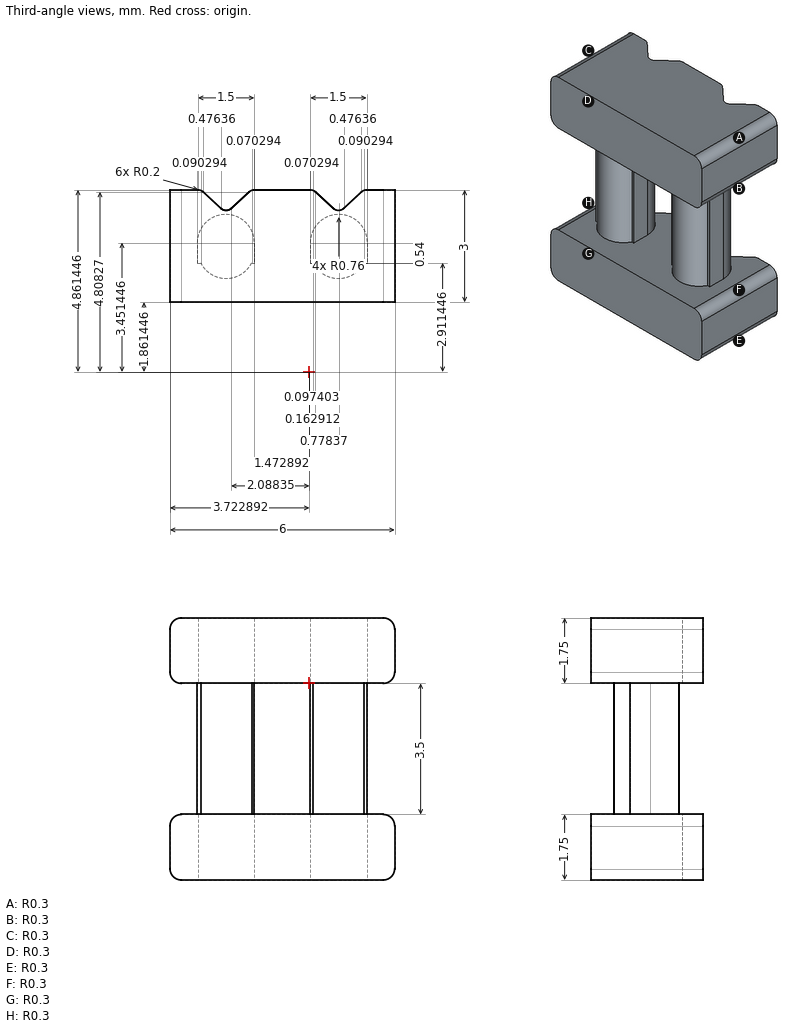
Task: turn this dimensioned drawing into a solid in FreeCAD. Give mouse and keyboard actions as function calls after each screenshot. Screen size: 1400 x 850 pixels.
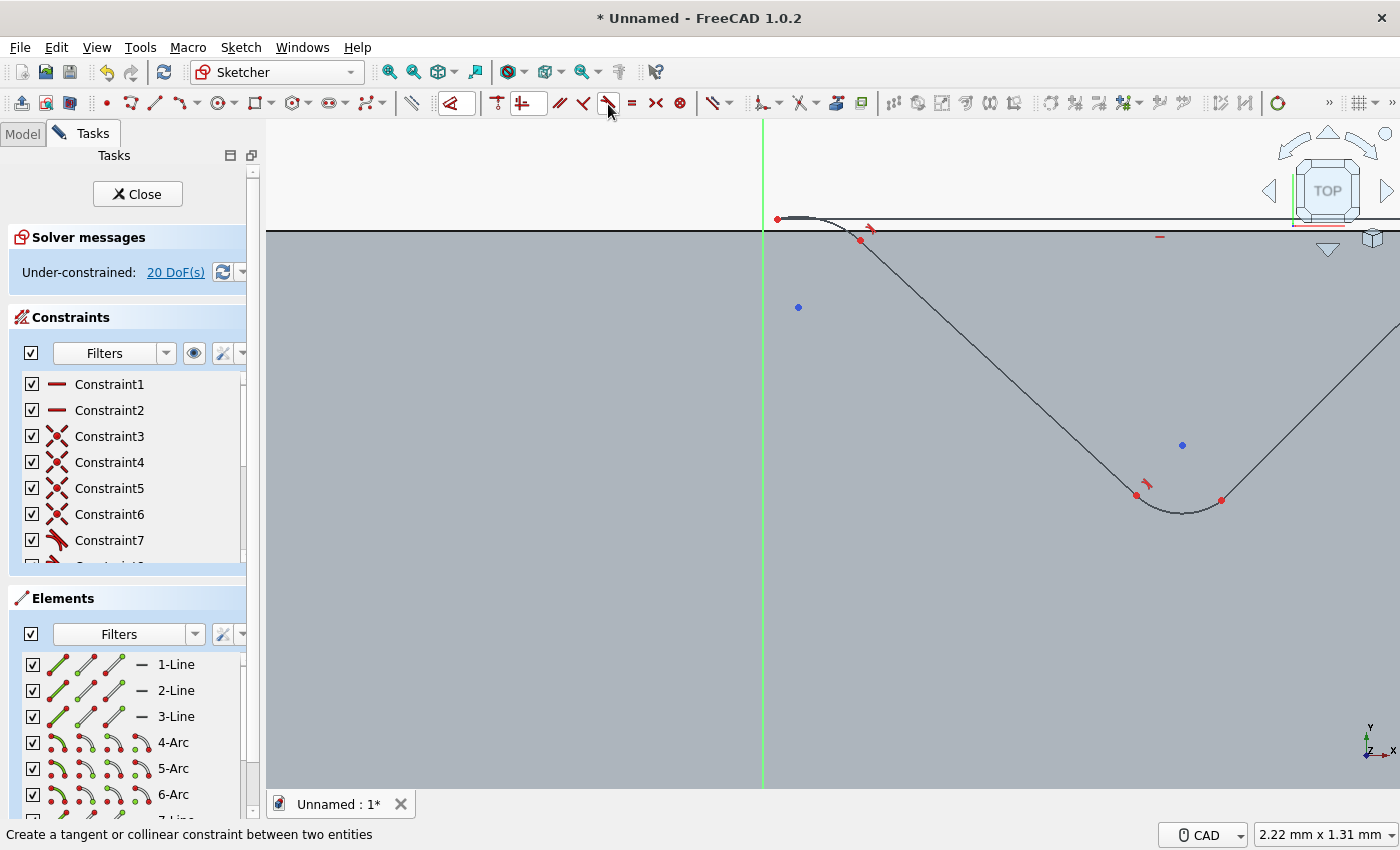
scroll(838, 252, down, 9)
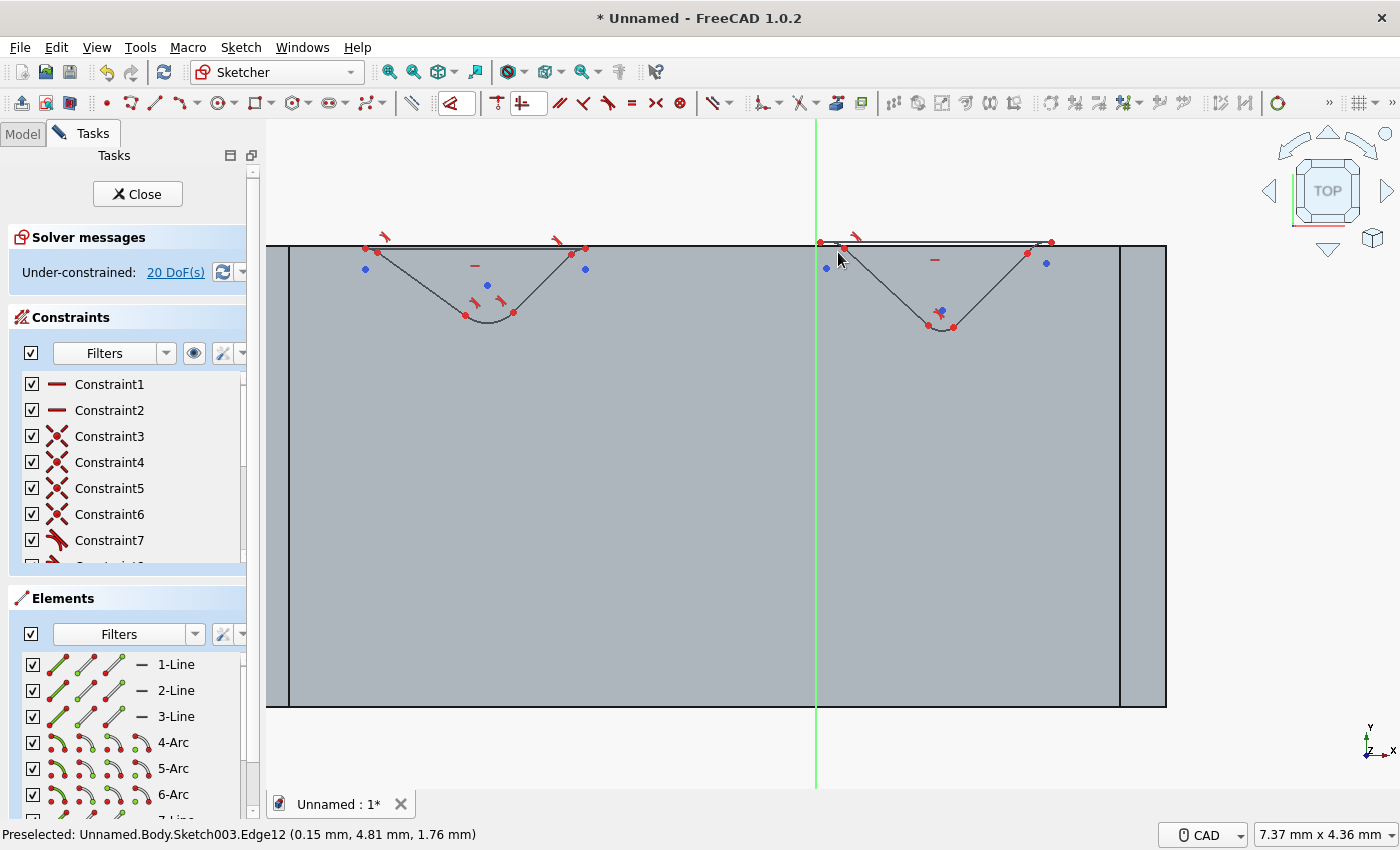
click(914, 281)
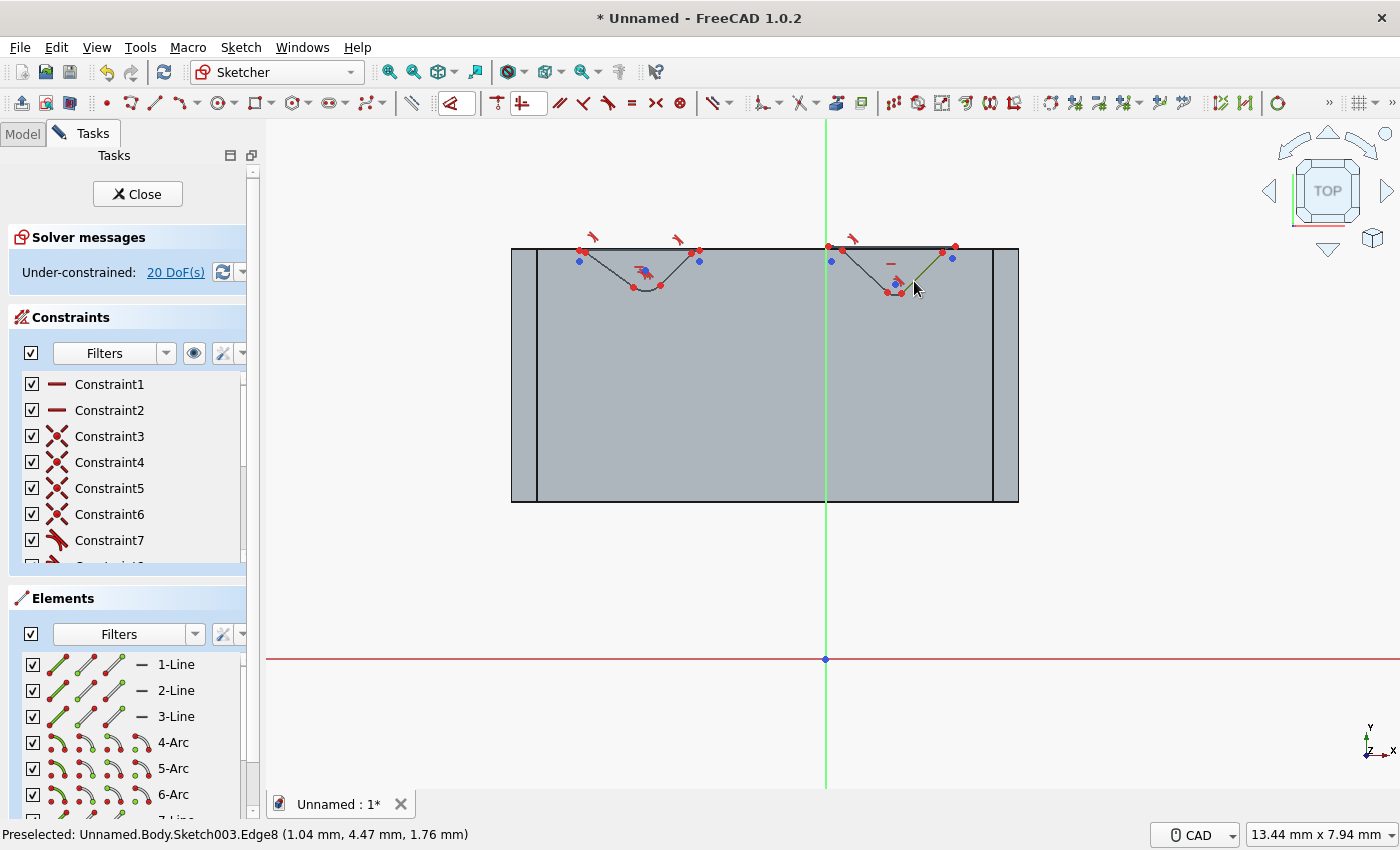
scroll(895, 295, up, 4)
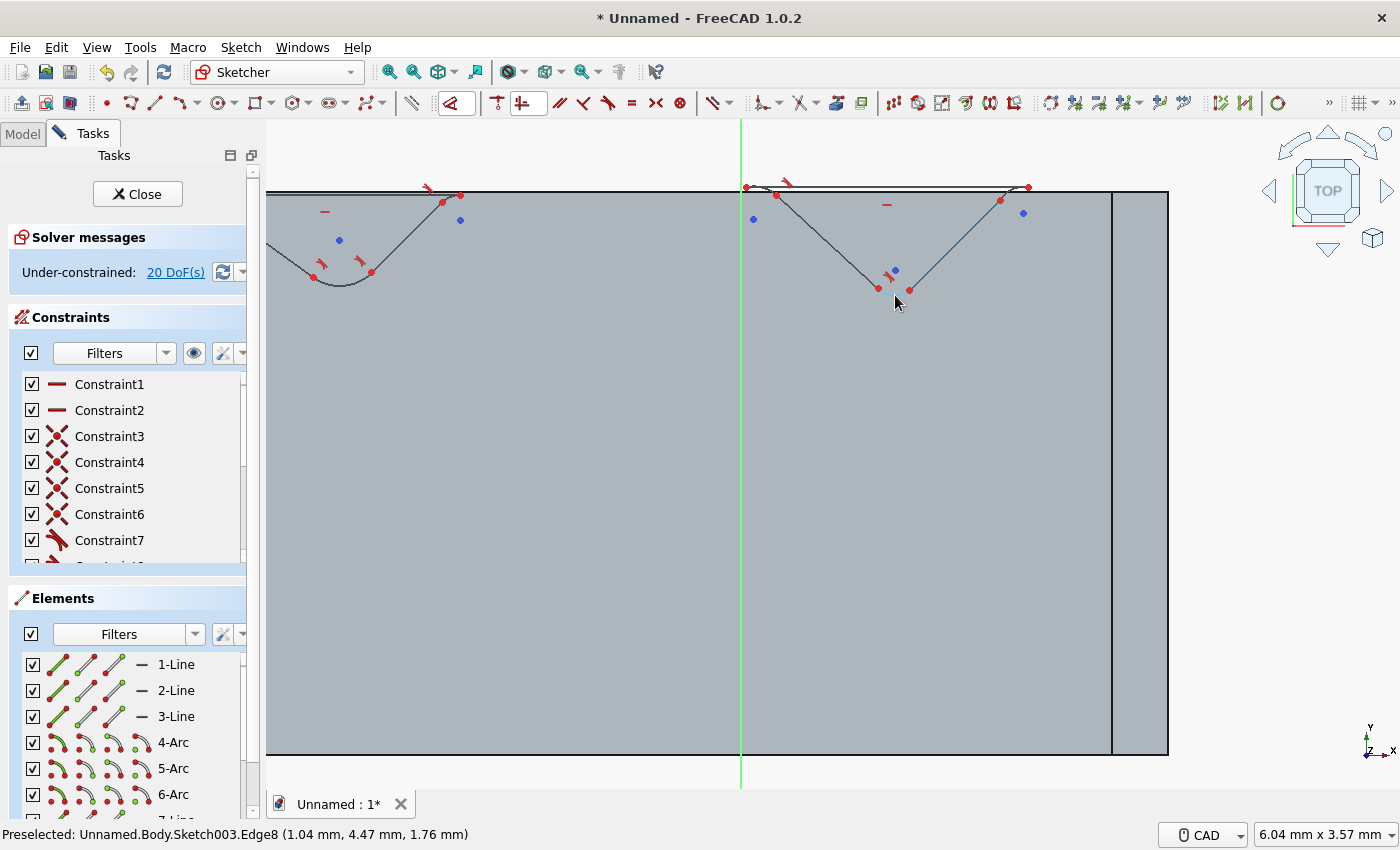
click(894, 296)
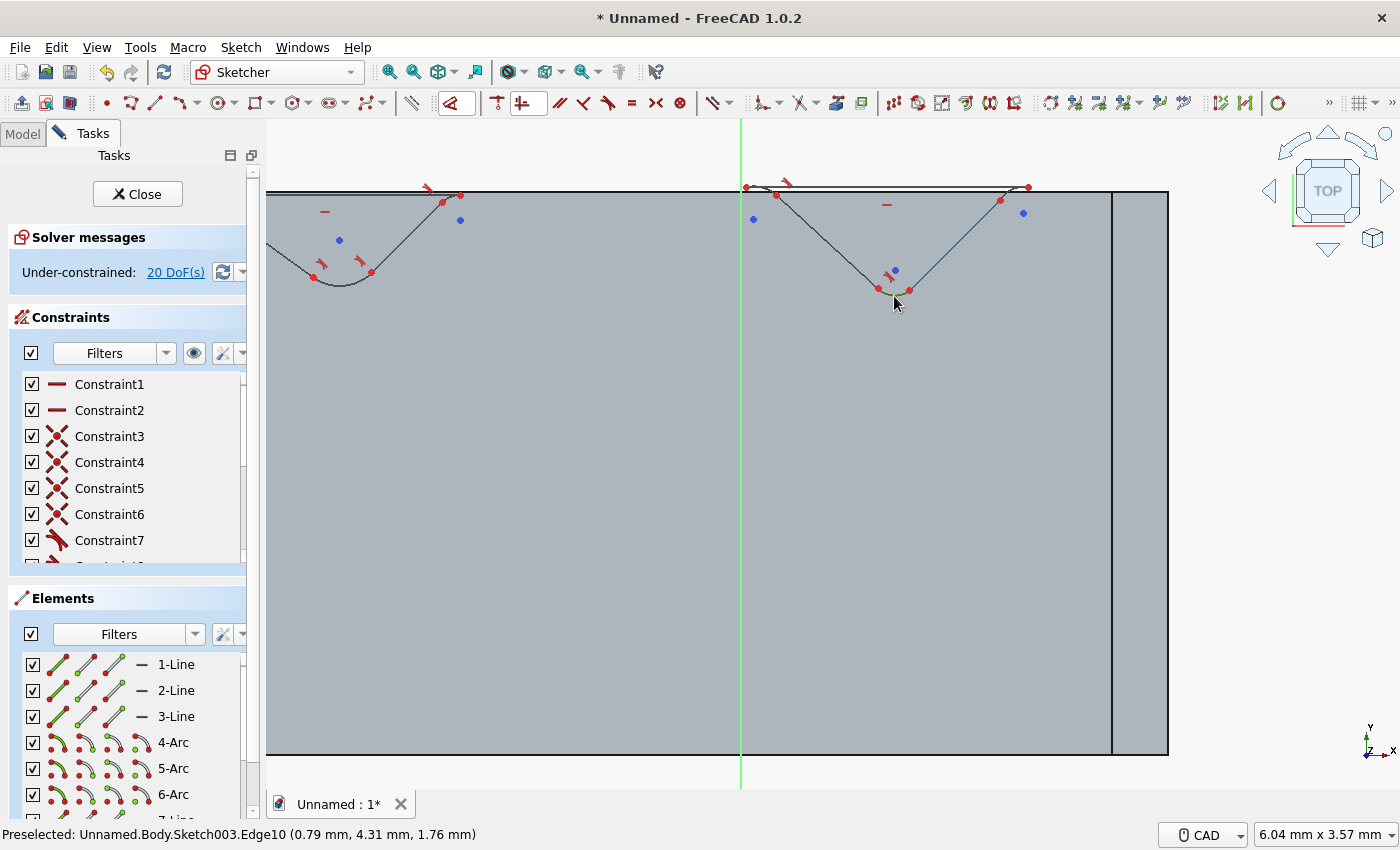
click(608, 104)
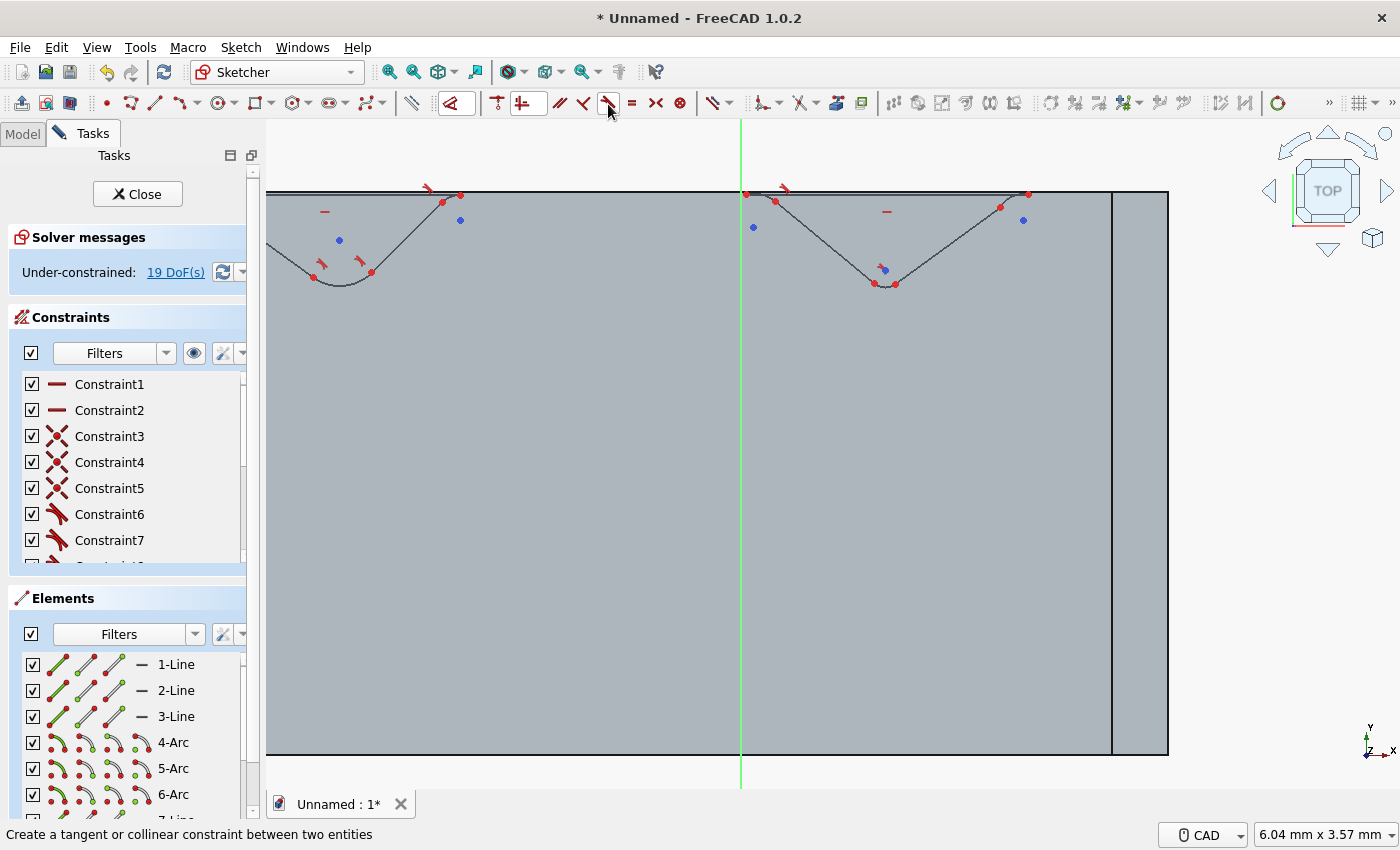
click(927, 261)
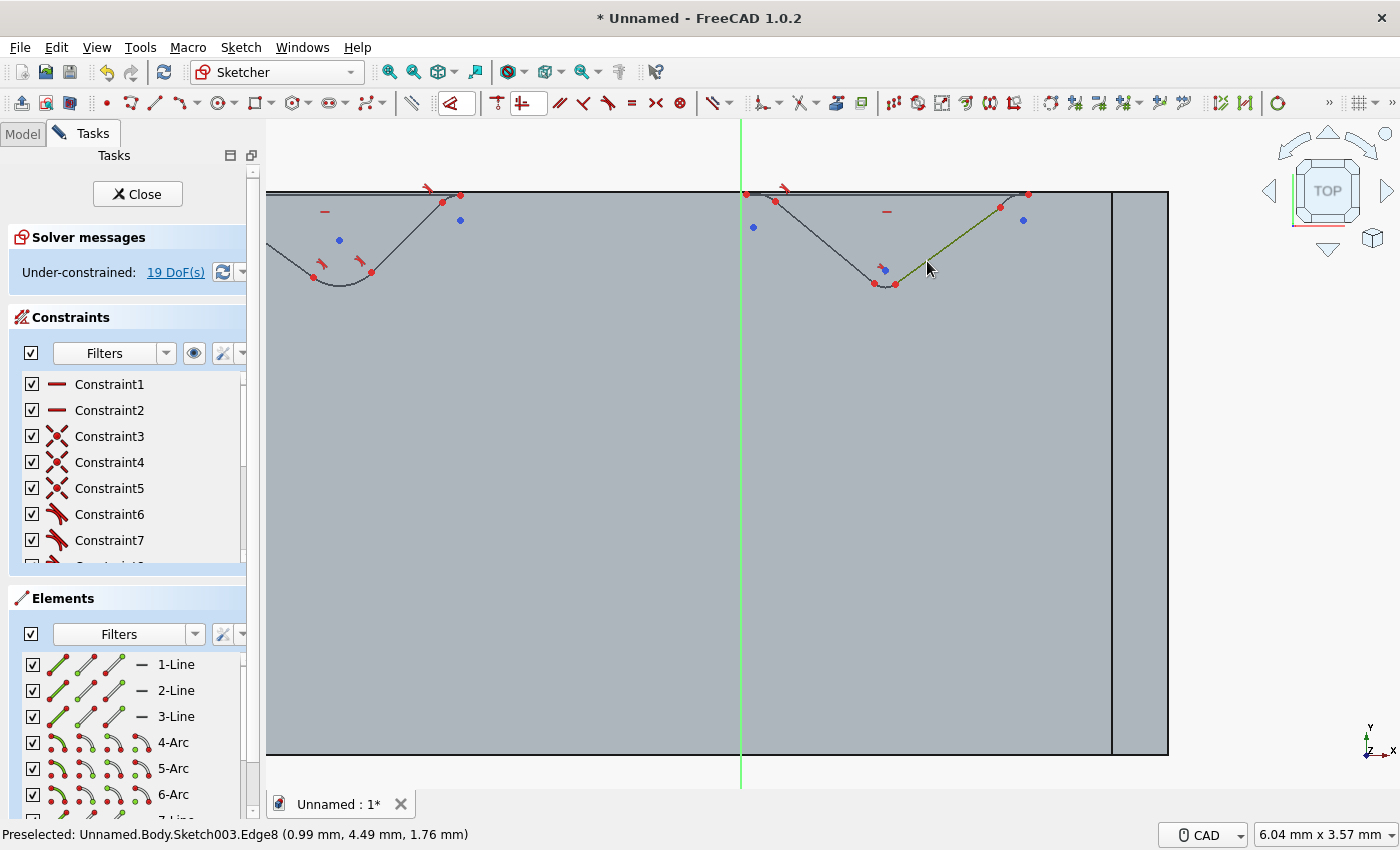
scroll(1004, 202, up, 4)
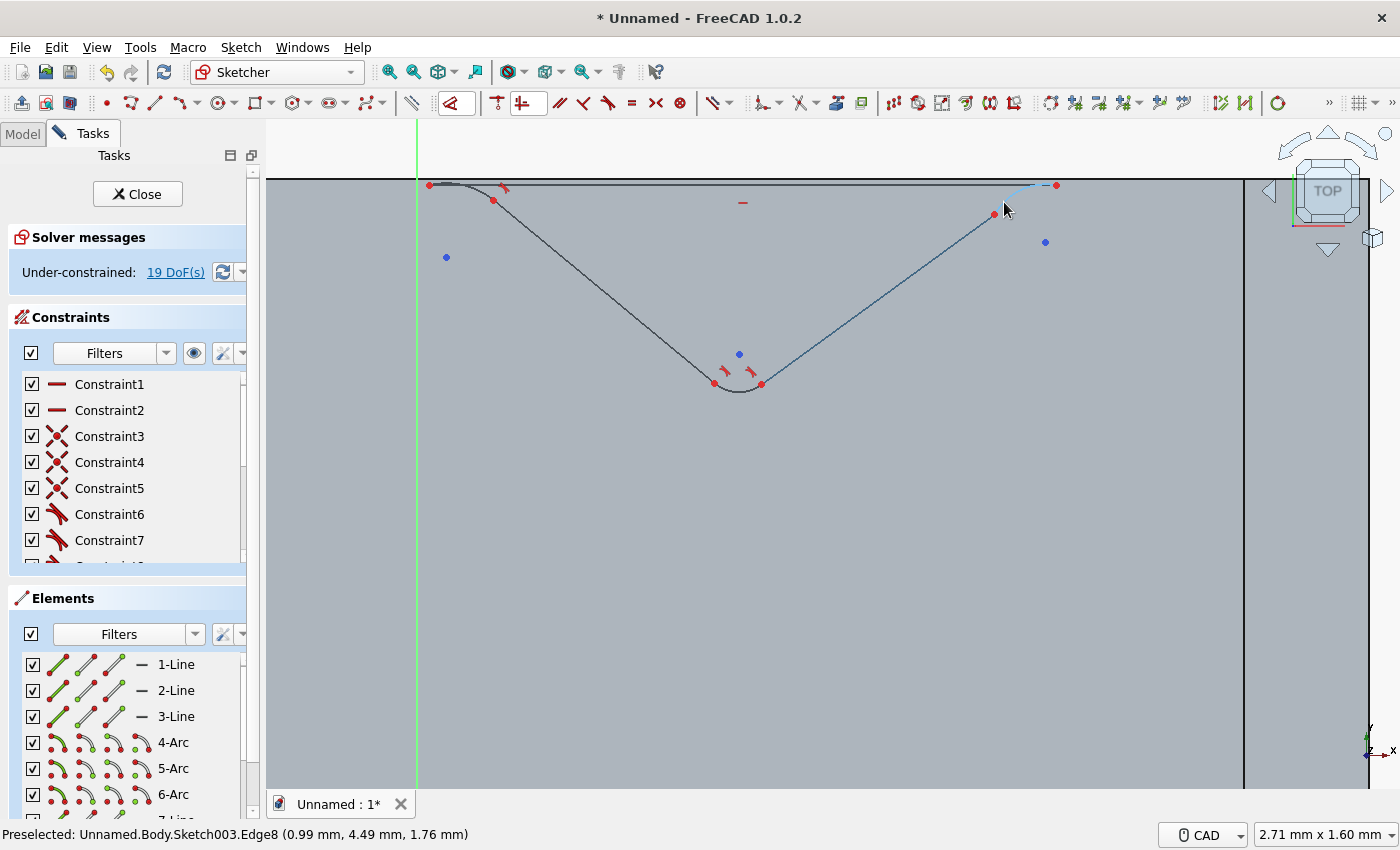
click(1003, 203)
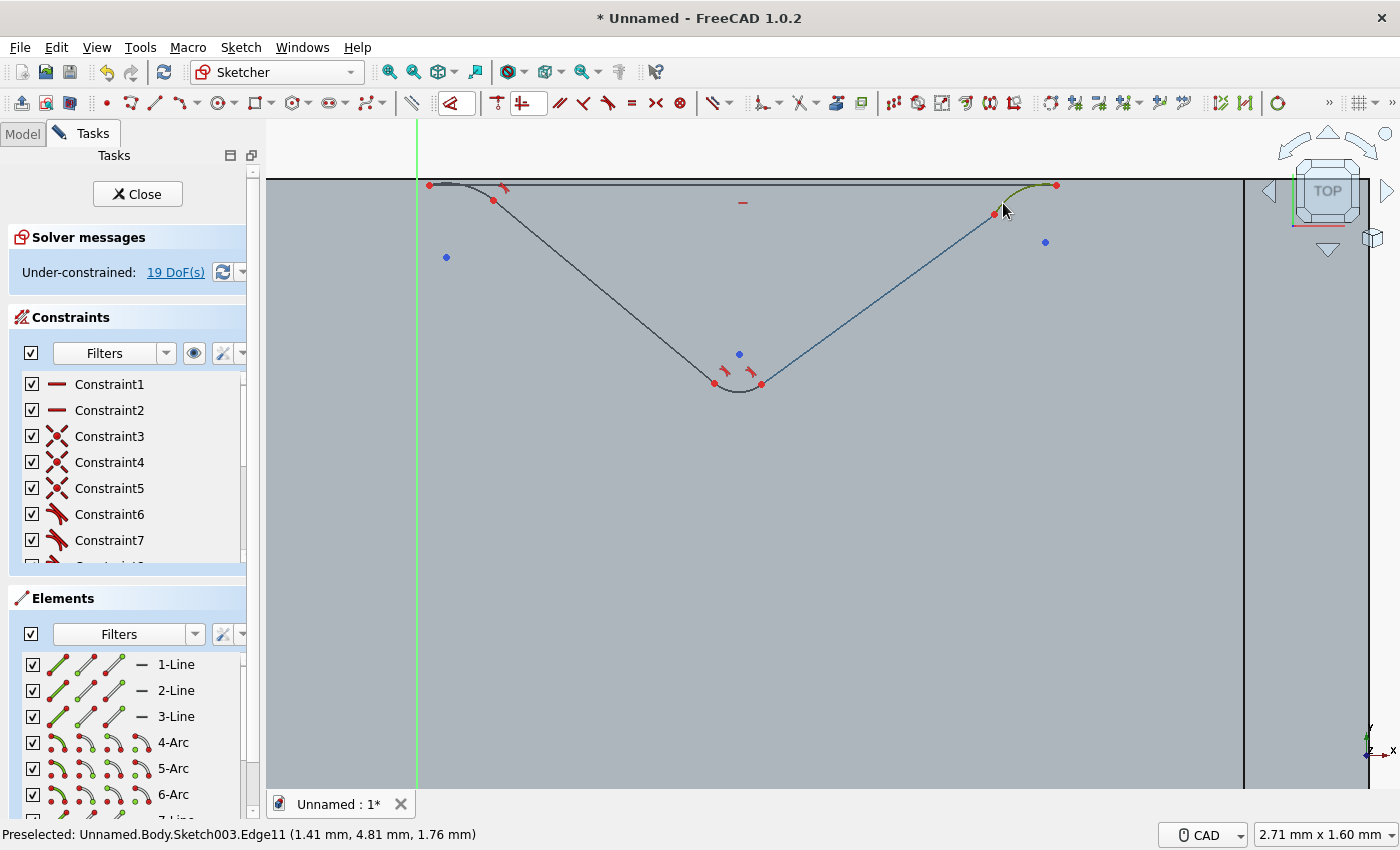
click(608, 104)